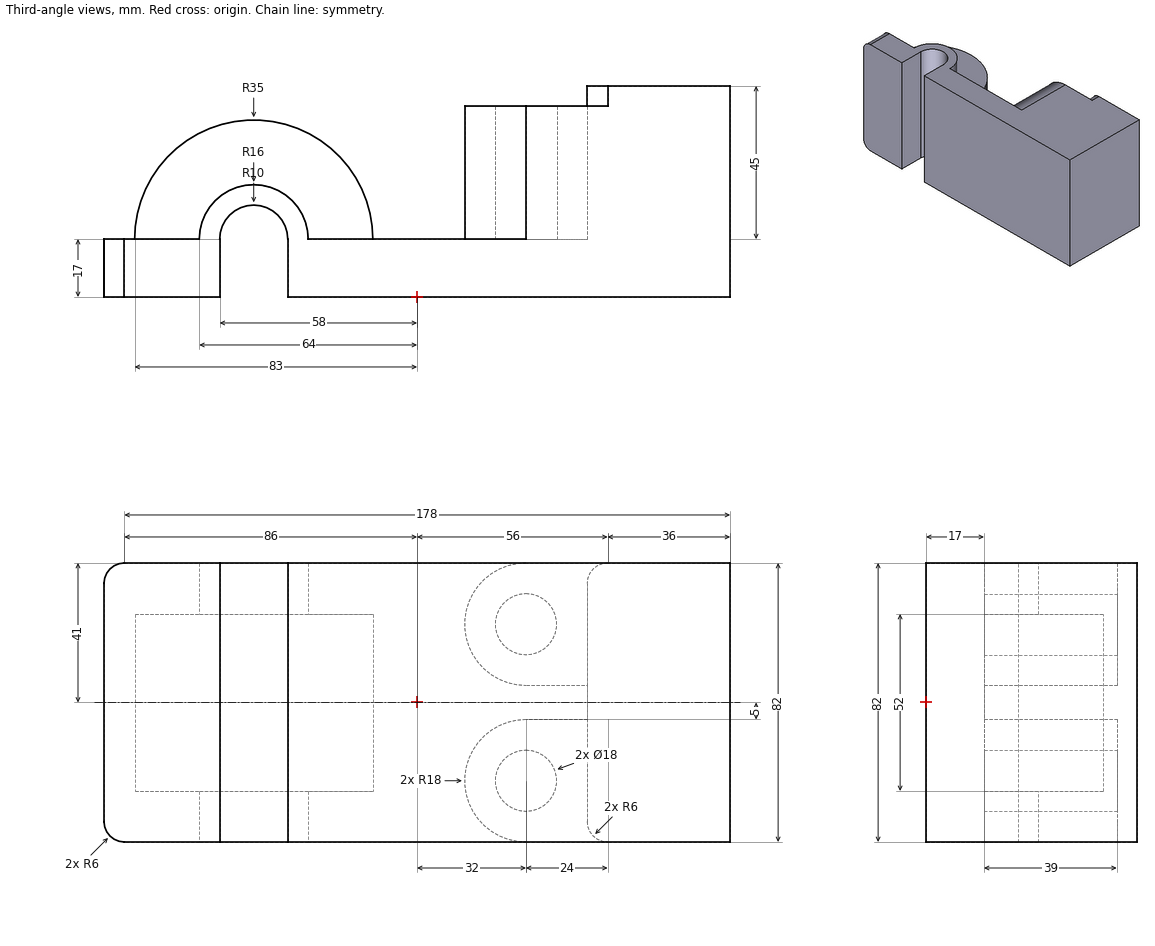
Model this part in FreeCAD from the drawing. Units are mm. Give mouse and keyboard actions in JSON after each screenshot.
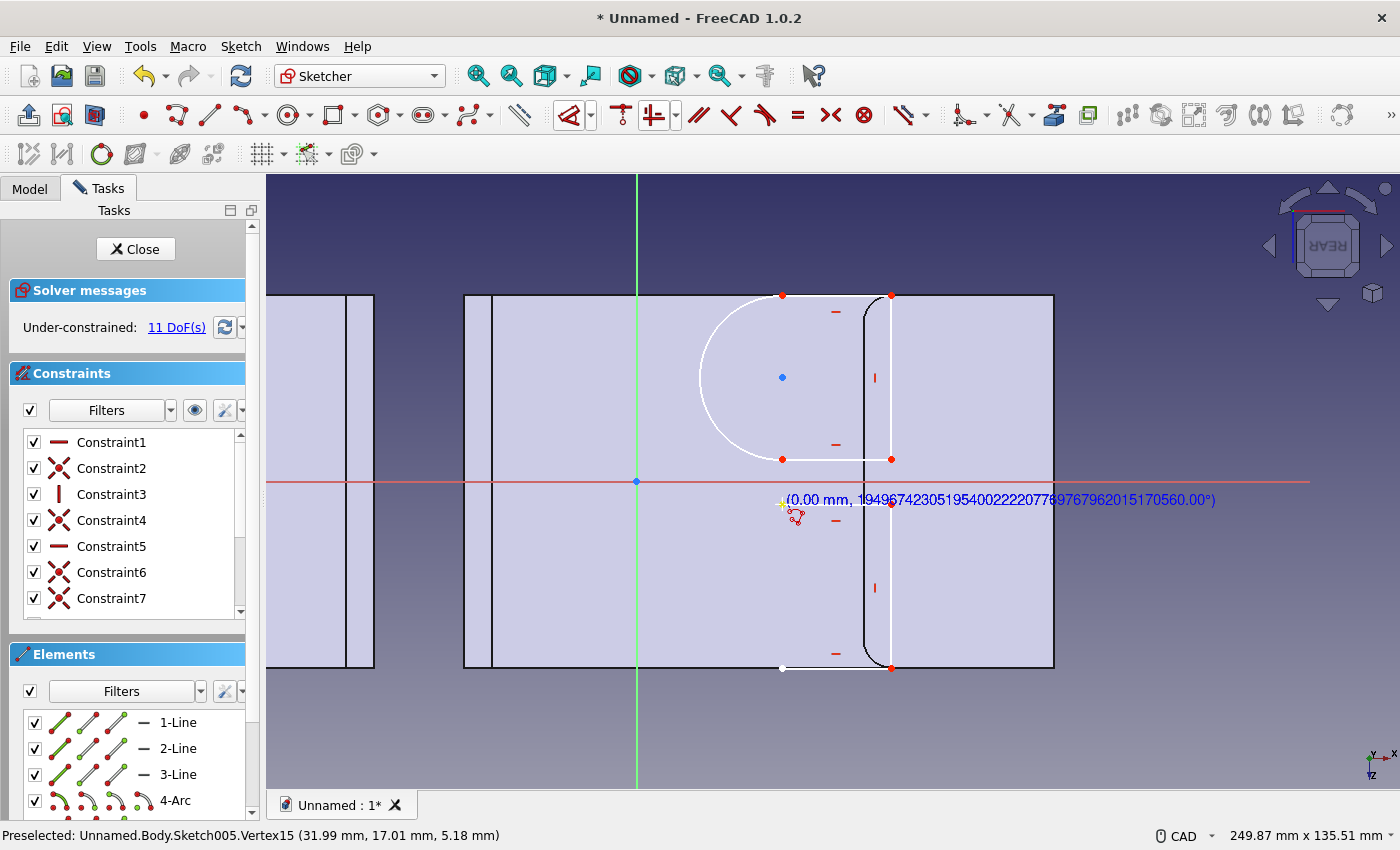
{"action": "left_click", "coordinate": [242, 116]}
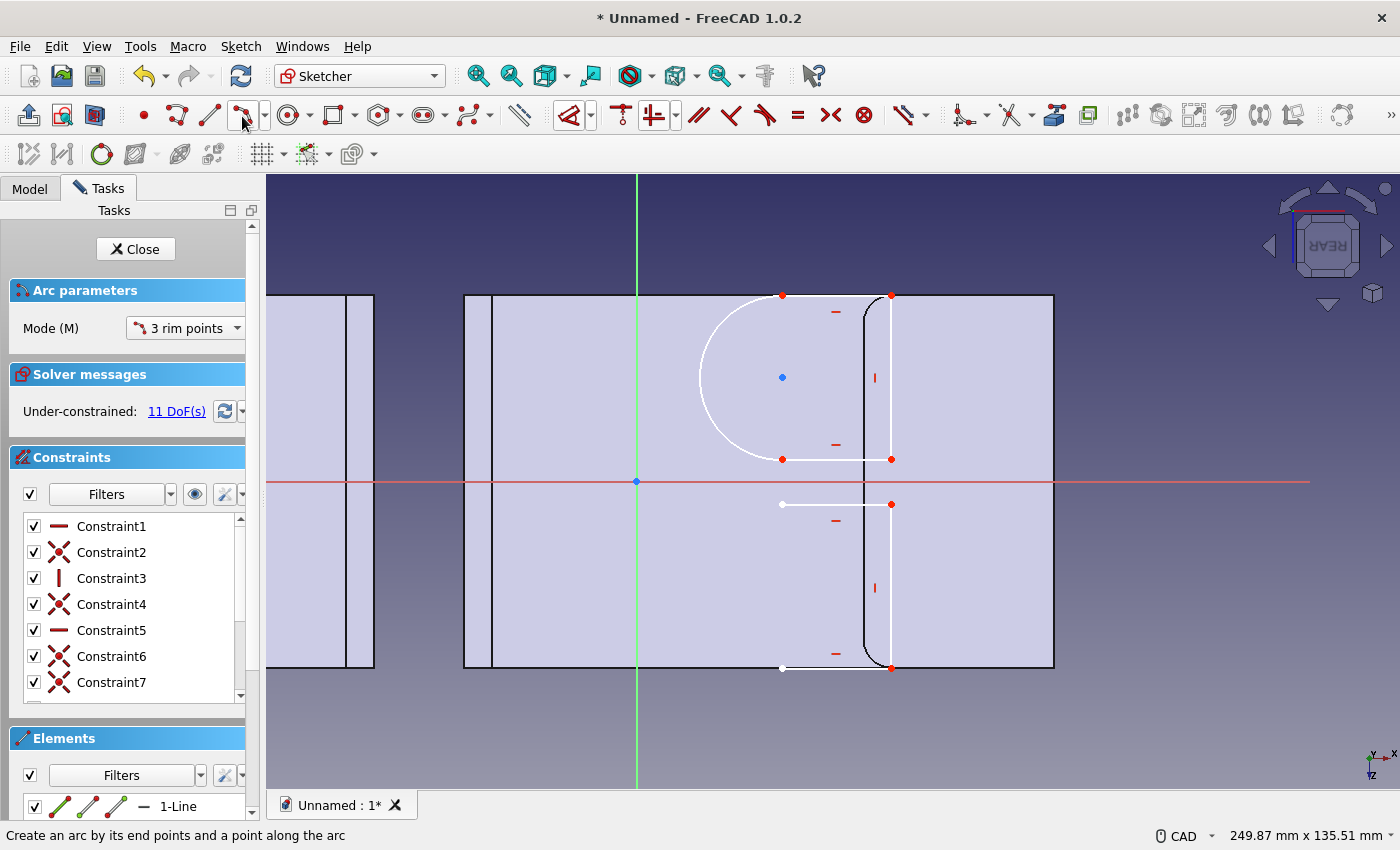
{"action": "left_click", "coordinate": [782, 505]}
{"action": "left_click", "coordinate": [782, 669]}
{"action": "left_click", "coordinate": [700, 586]}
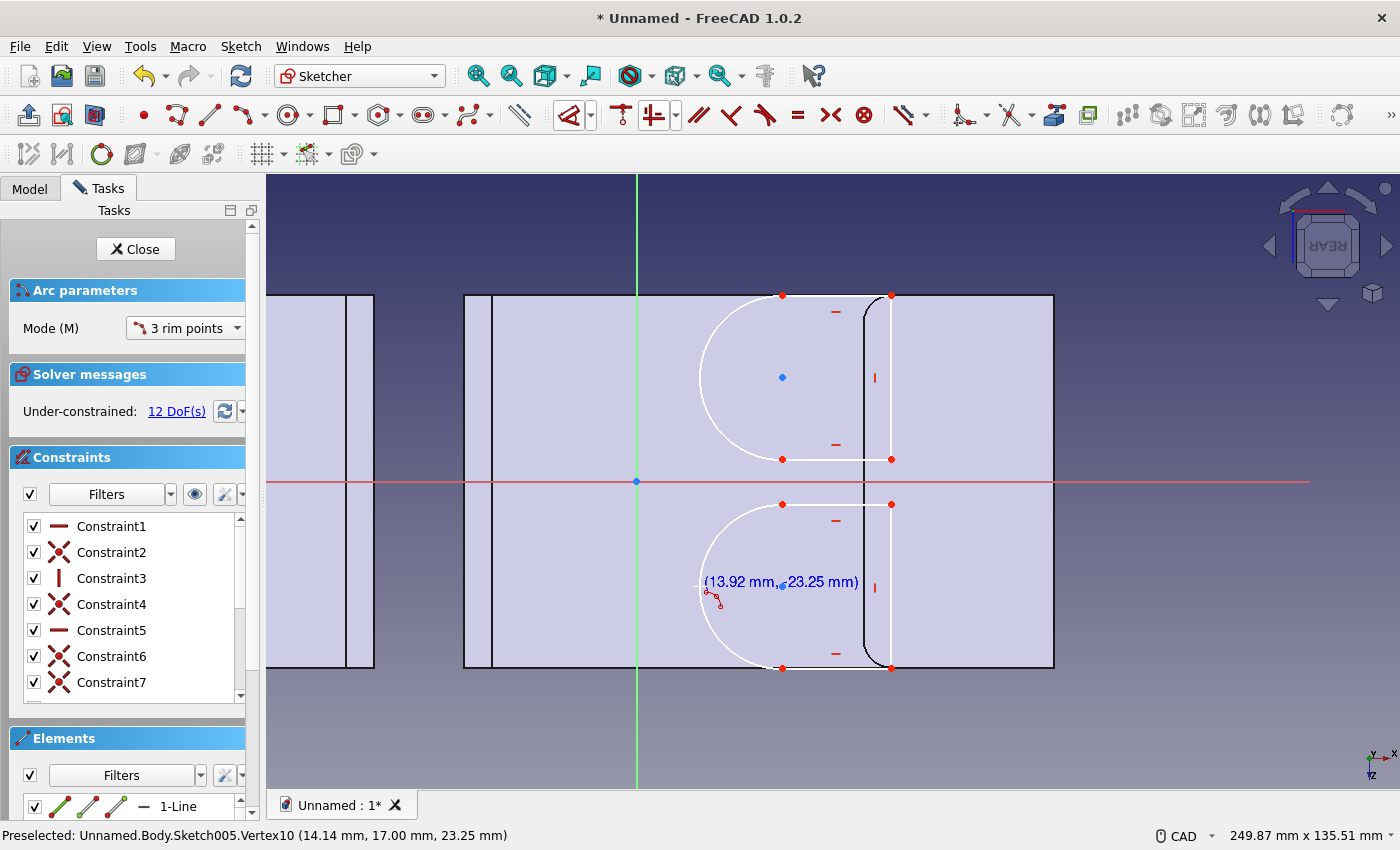
{"action": "left_click", "coordinate": [288, 116]}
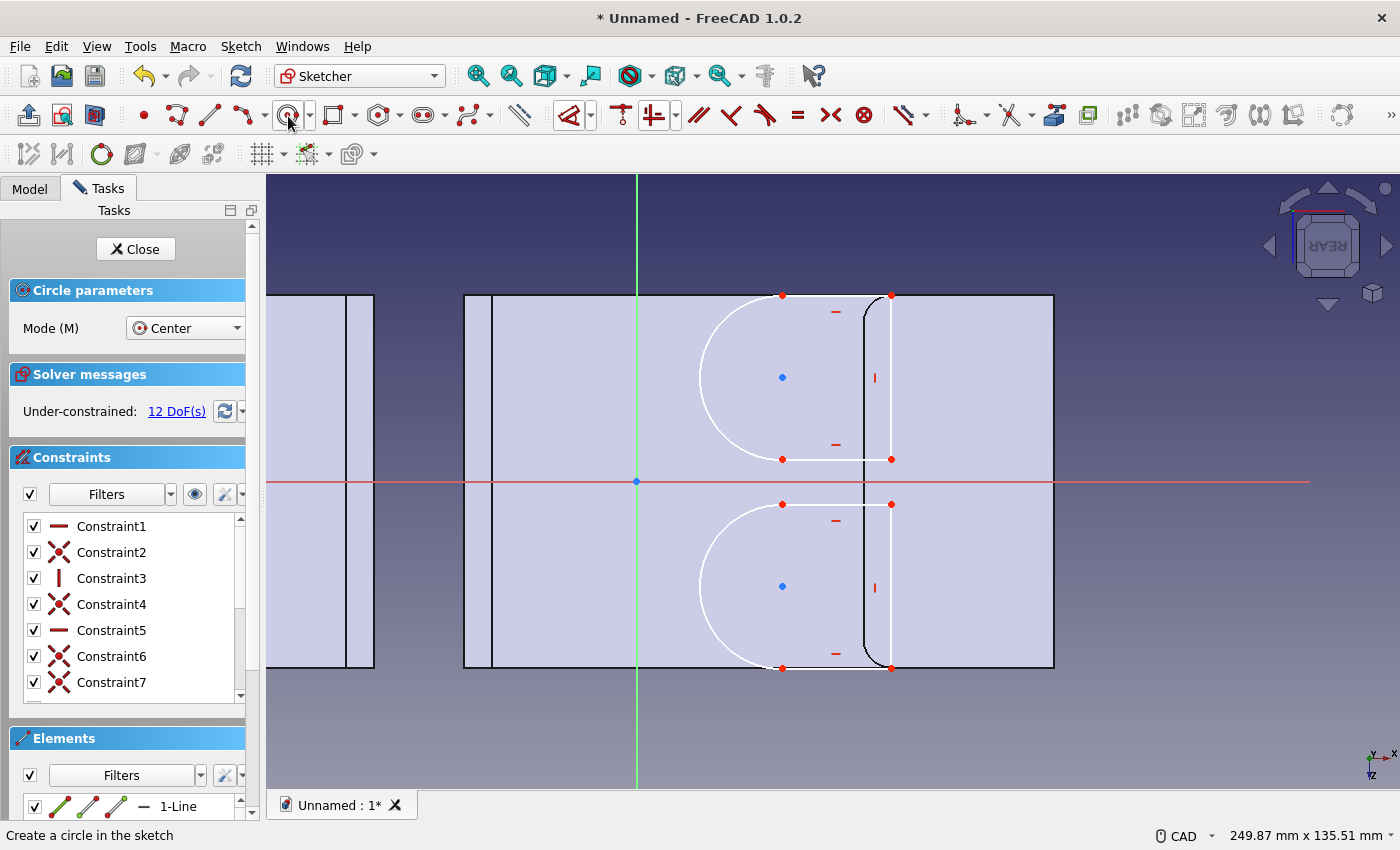
{"action": "left_click", "coordinate": [782, 377]}
{"action": "mouse_move", "coordinate": [811, 348]}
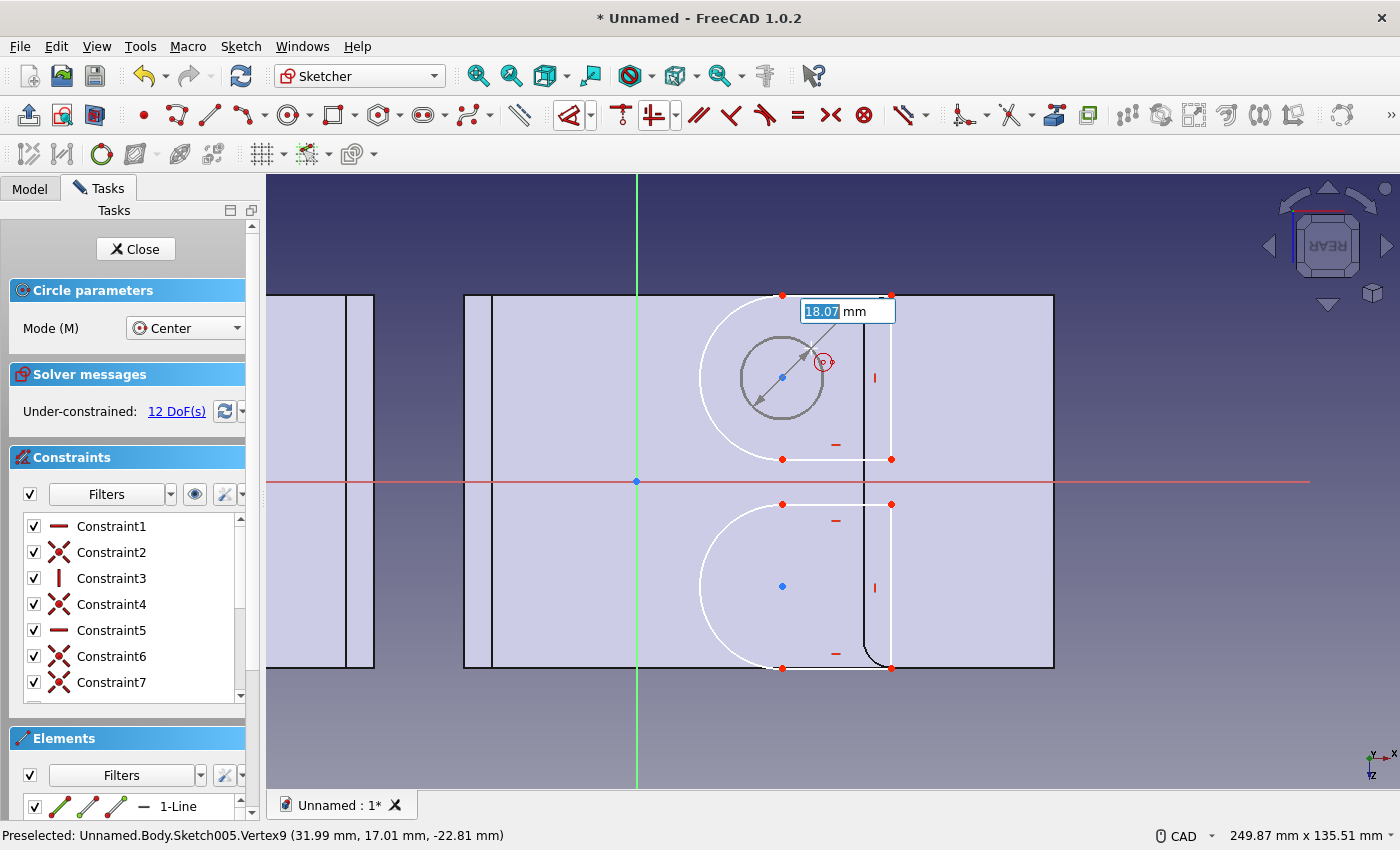
{"action": "type", "text": "18"}
{"action": "key", "text": "Return"}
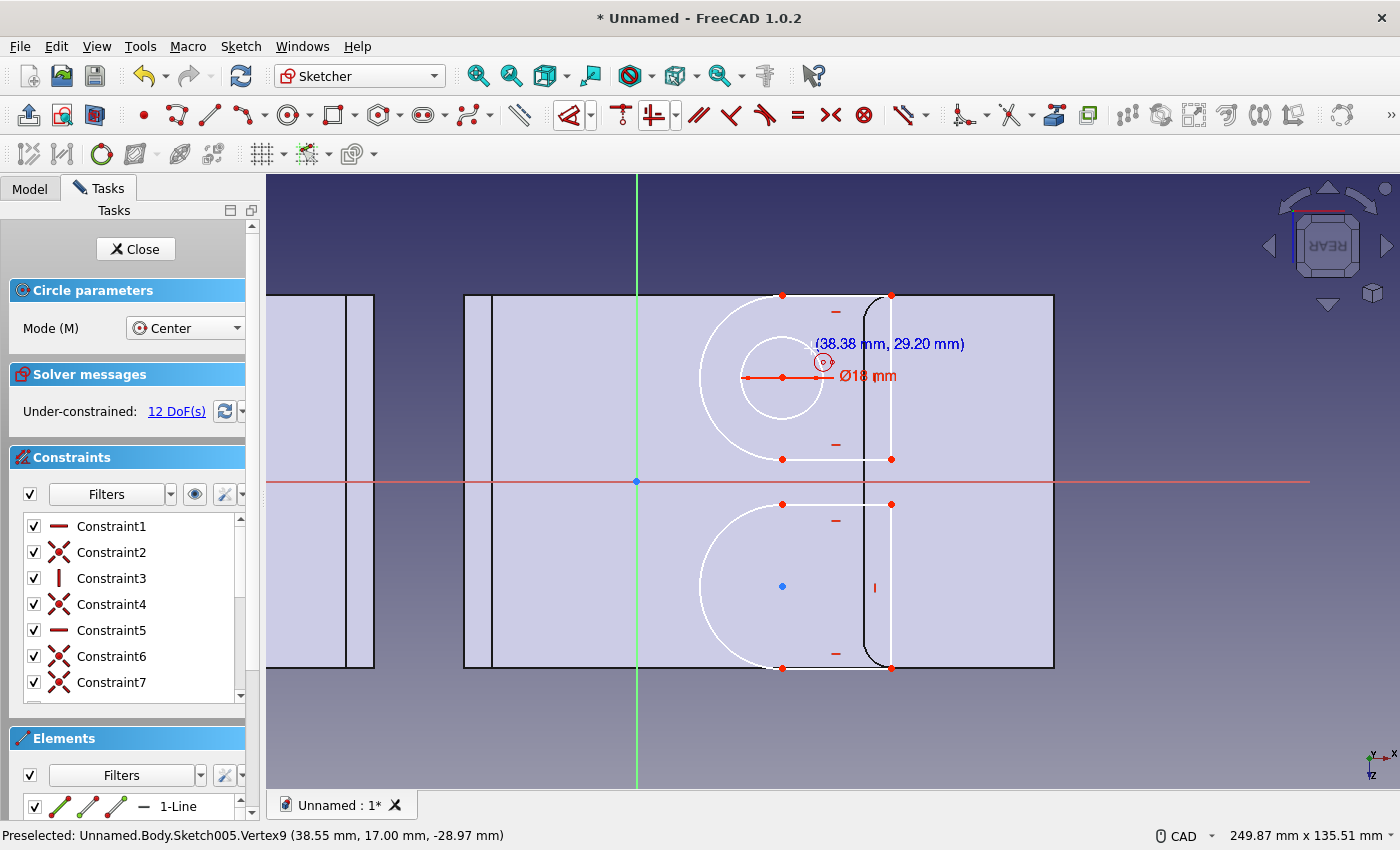
{"action": "left_click", "coordinate": [782, 586]}
{"action": "mouse_move", "coordinate": [811, 557]}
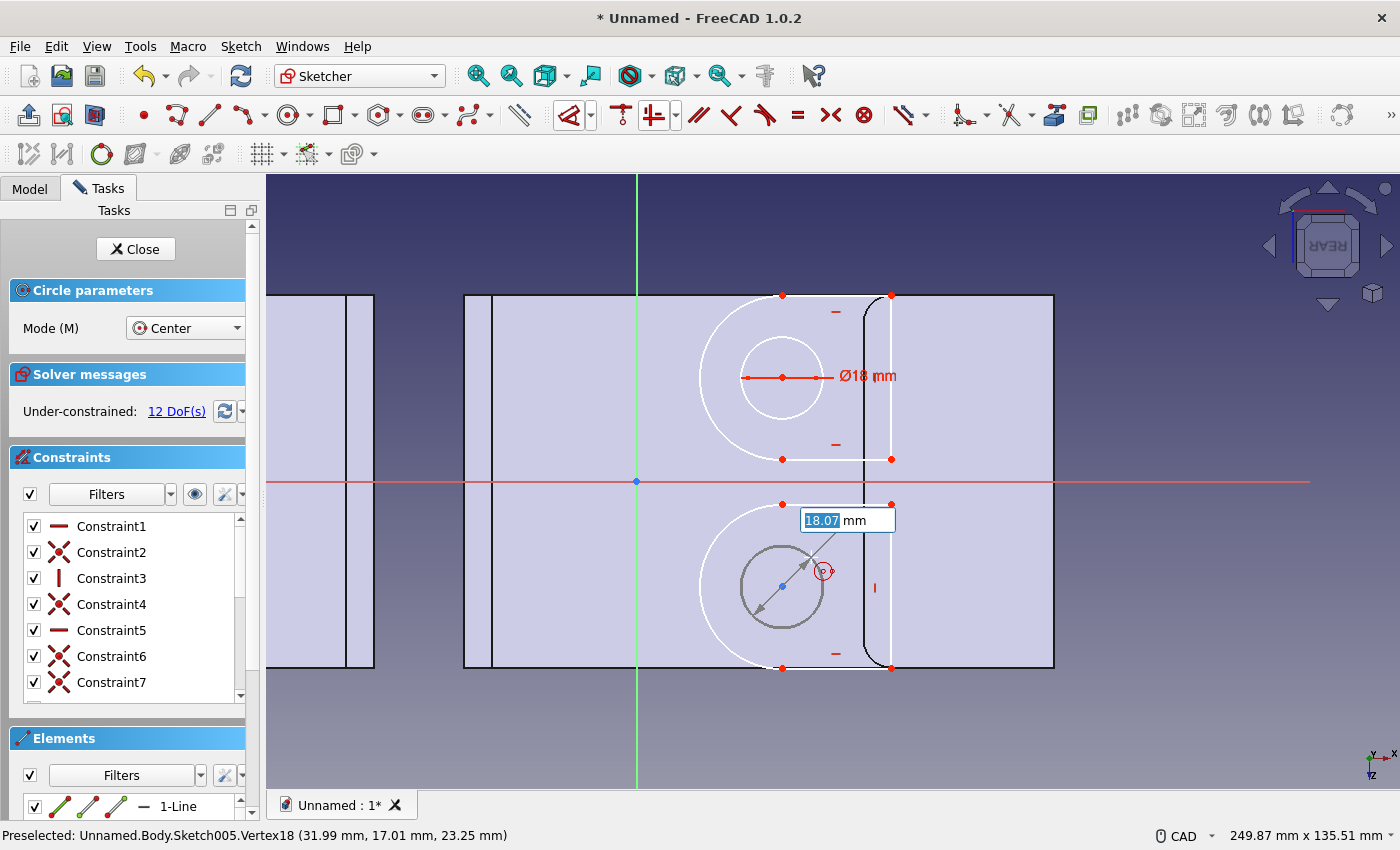
{"action": "type", "text": "18"}
{"action": "key", "text": "Return"}
{"action": "key", "text": "Escape"}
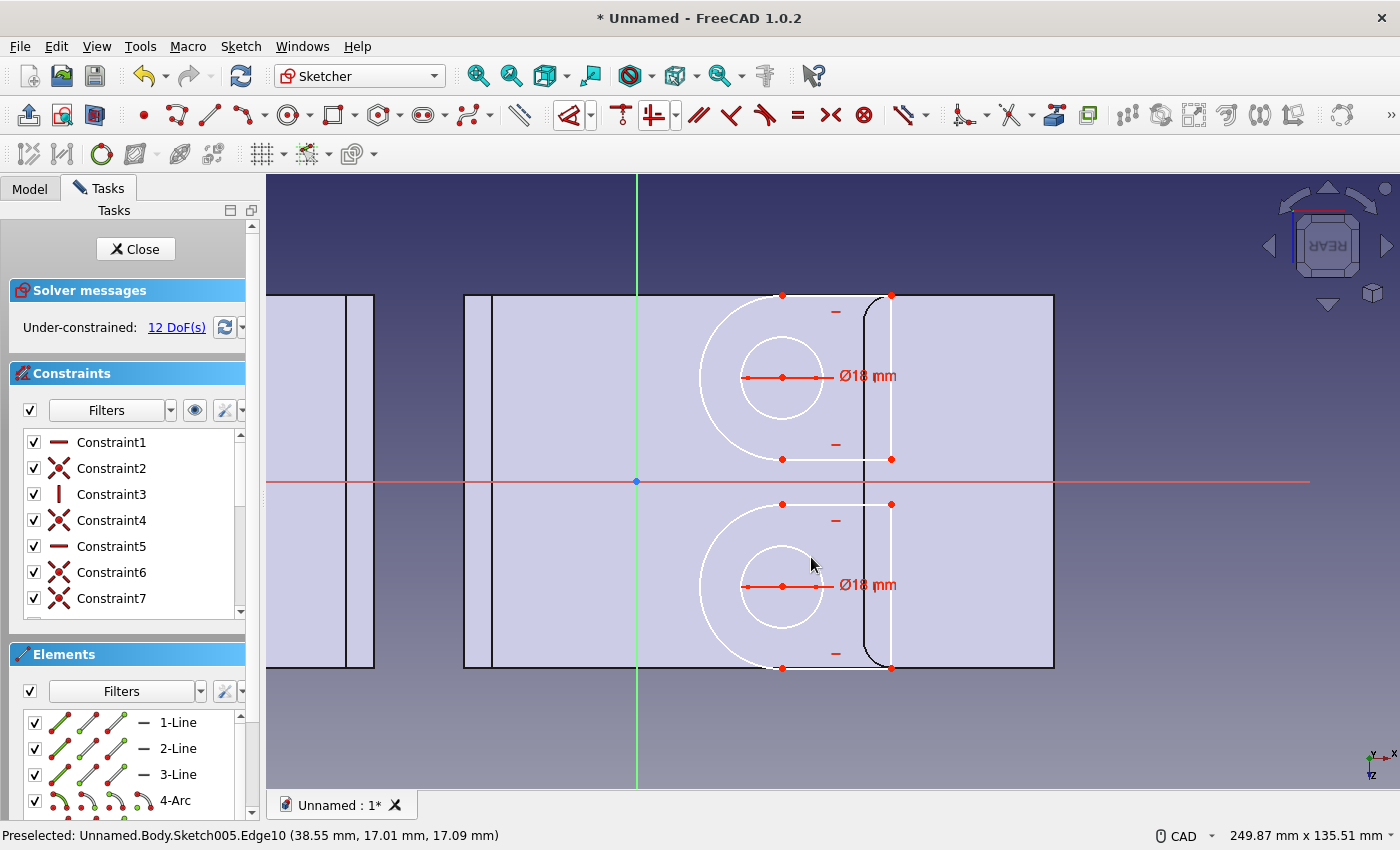
{"action": "left_click", "coordinate": [815, 460]}